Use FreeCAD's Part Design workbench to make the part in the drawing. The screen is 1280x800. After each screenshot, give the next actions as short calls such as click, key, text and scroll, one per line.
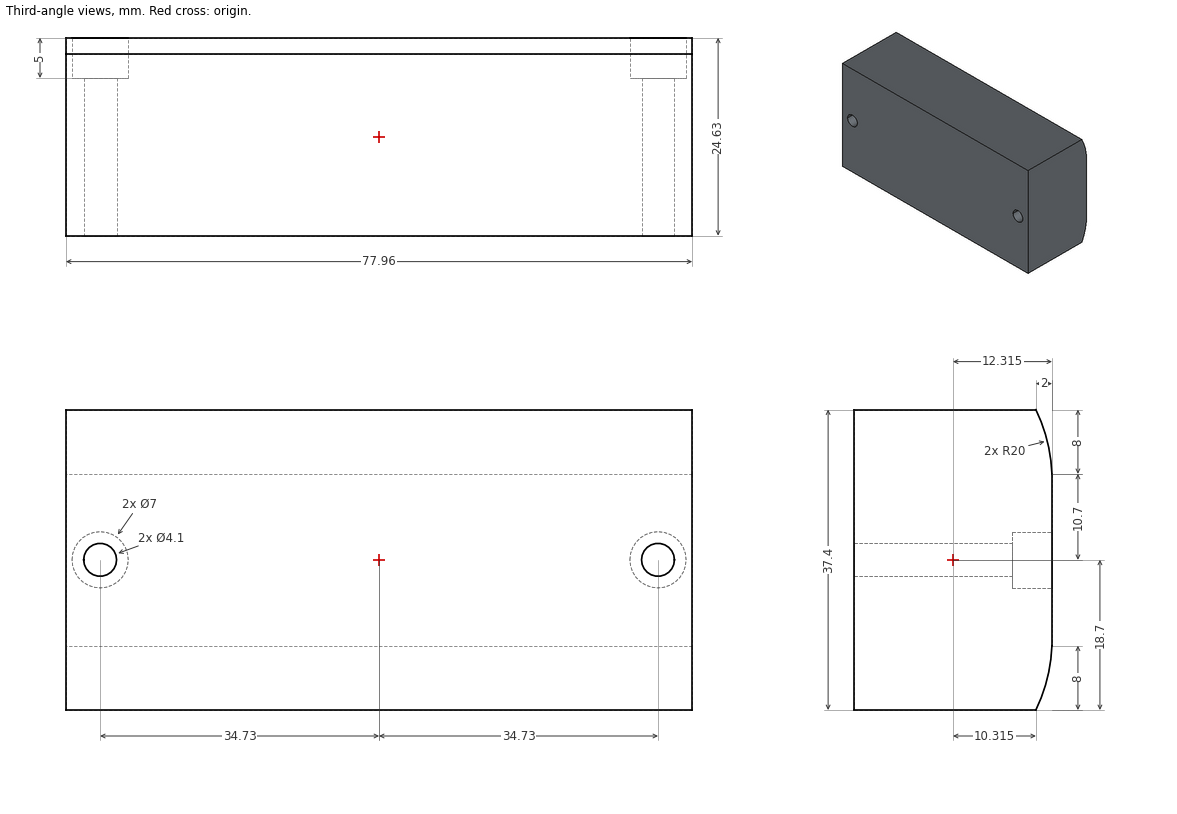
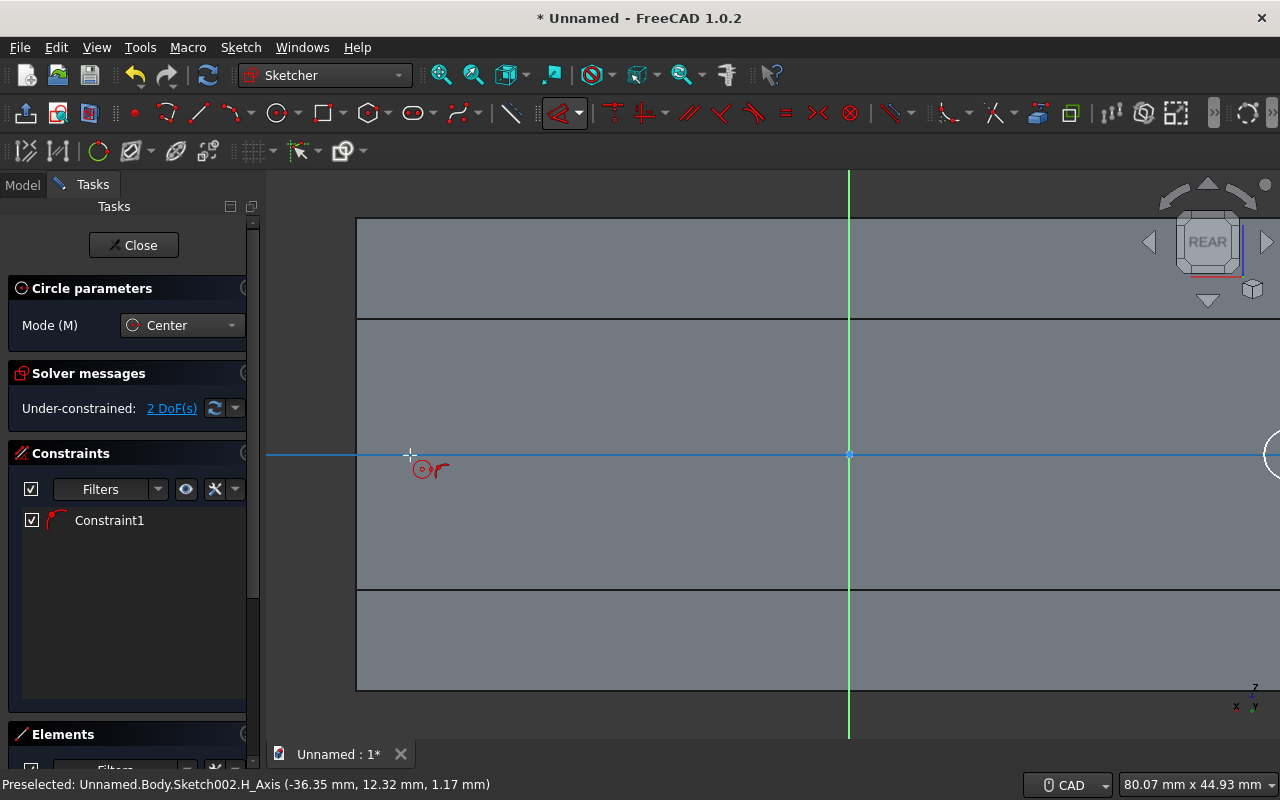
click(410, 454)
click(428, 436)
key(Escape)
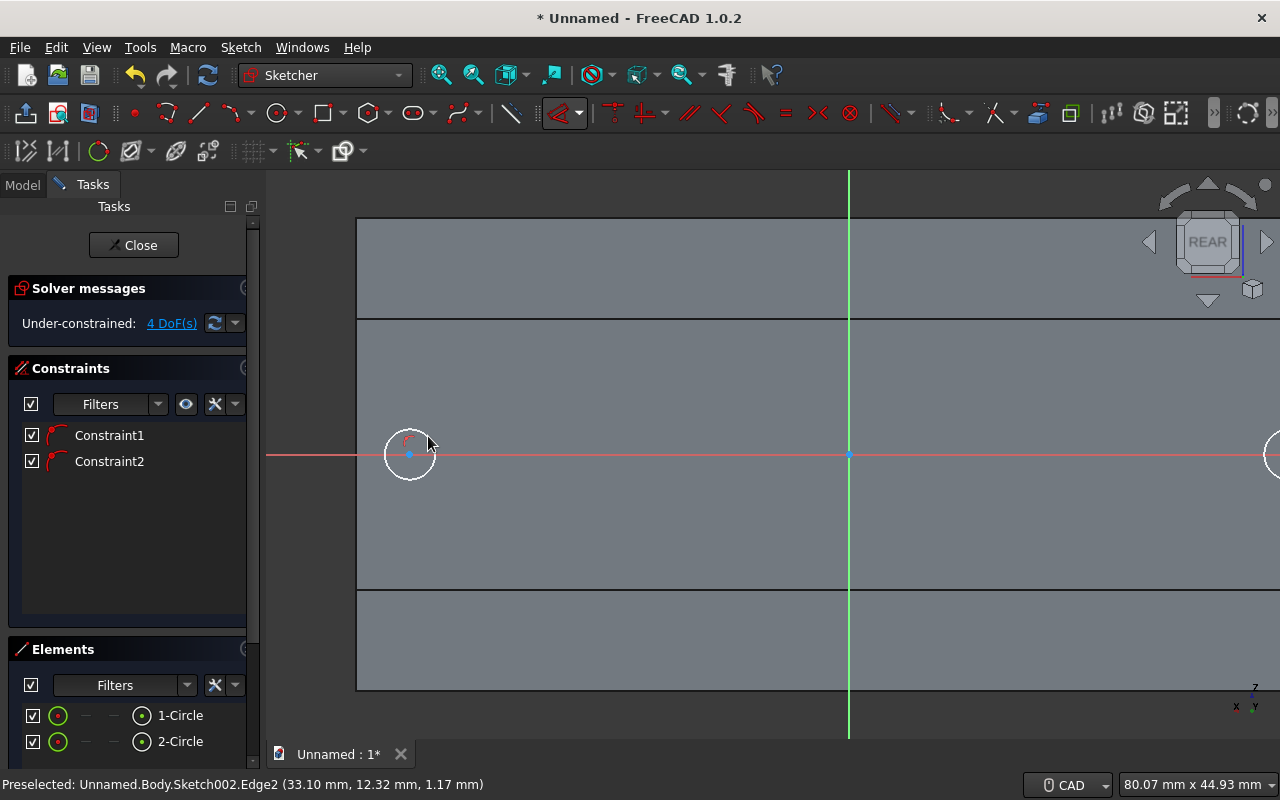
scroll(410, 455, down, 2)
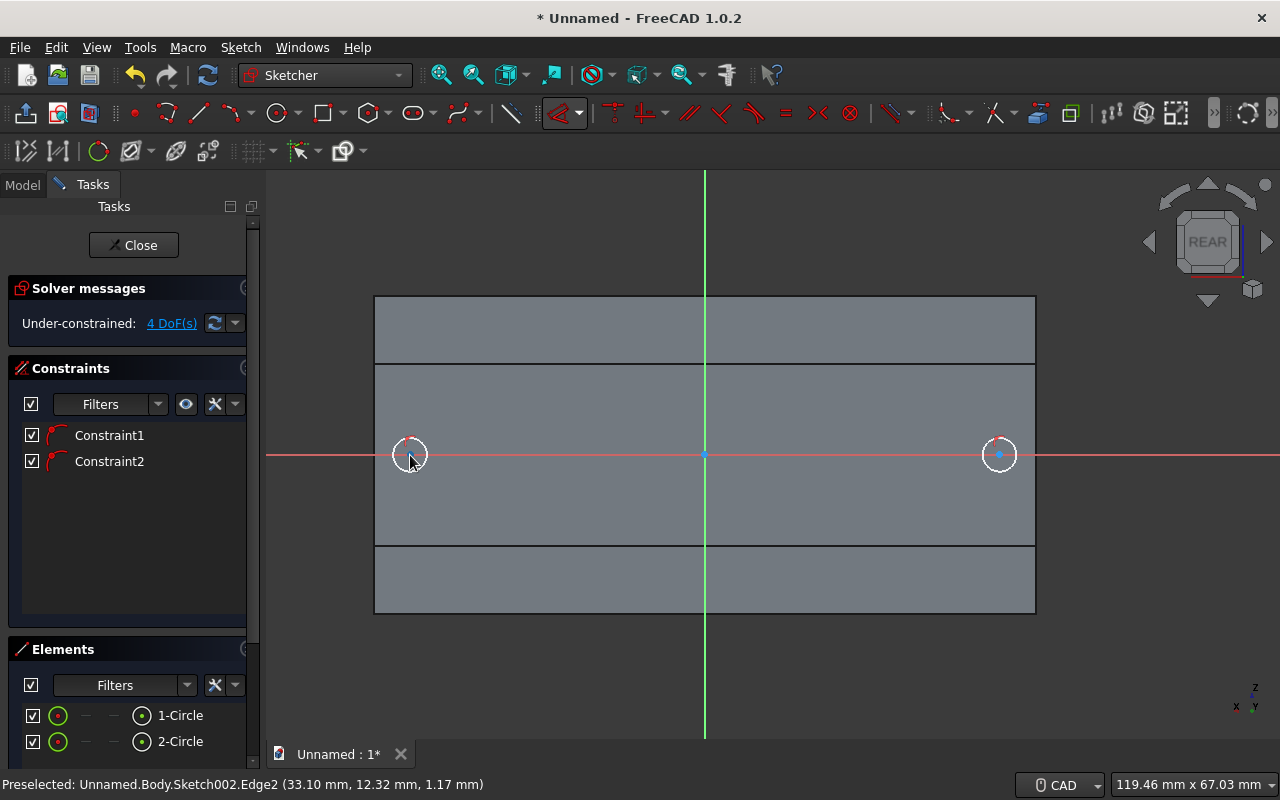
click(1011, 443)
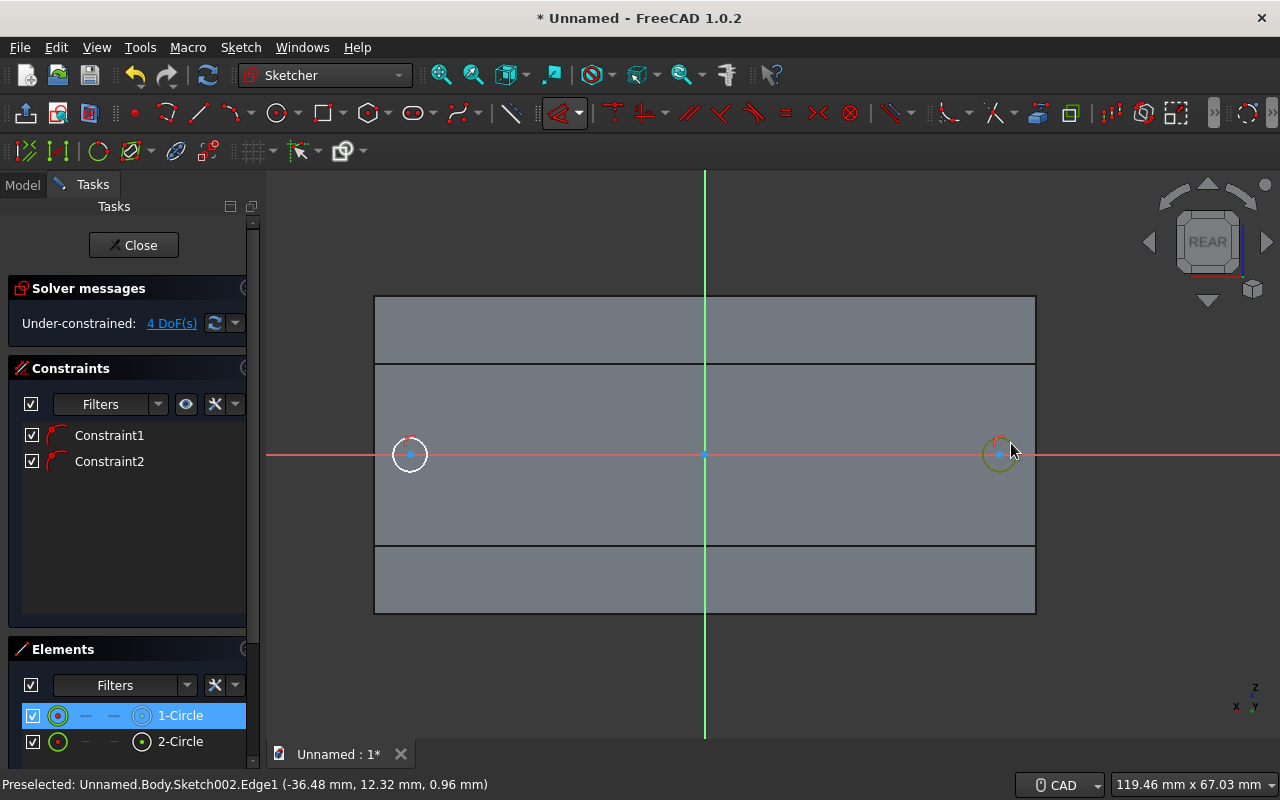
click(422, 443)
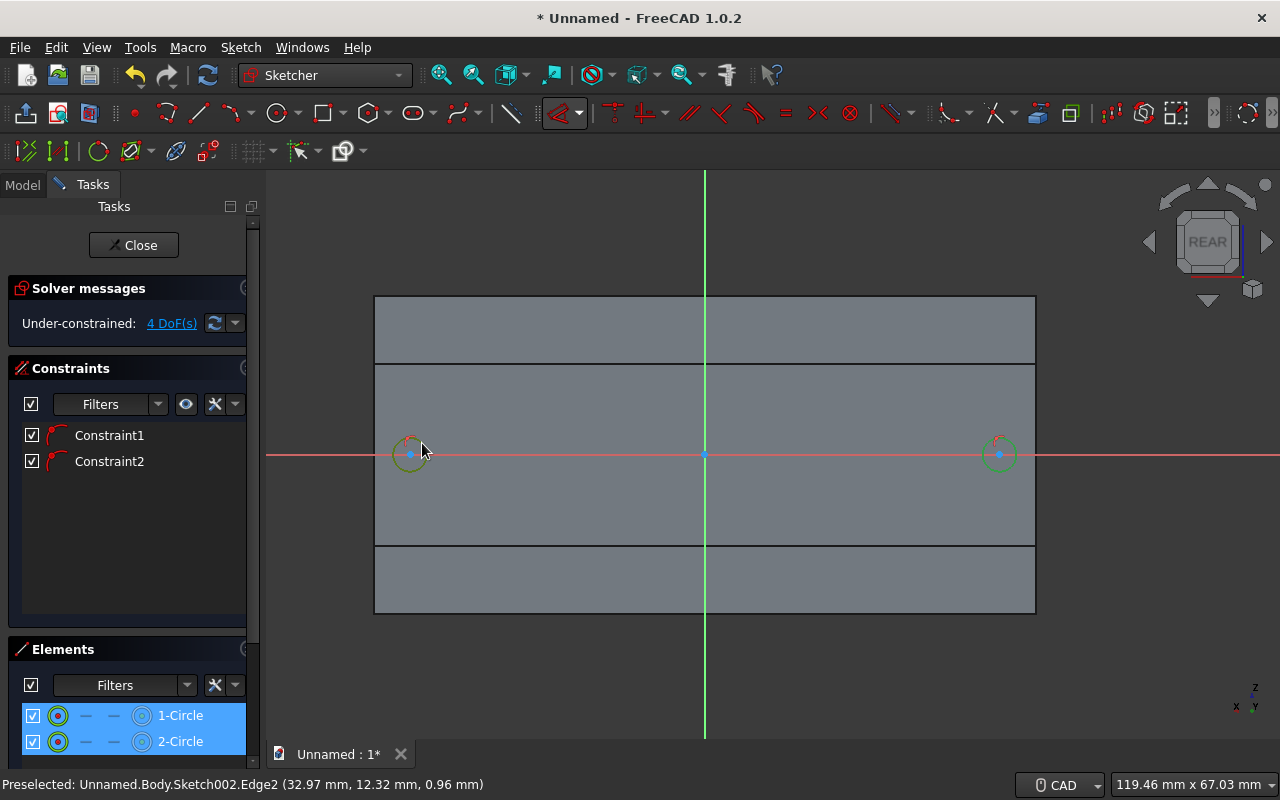
click(786, 114)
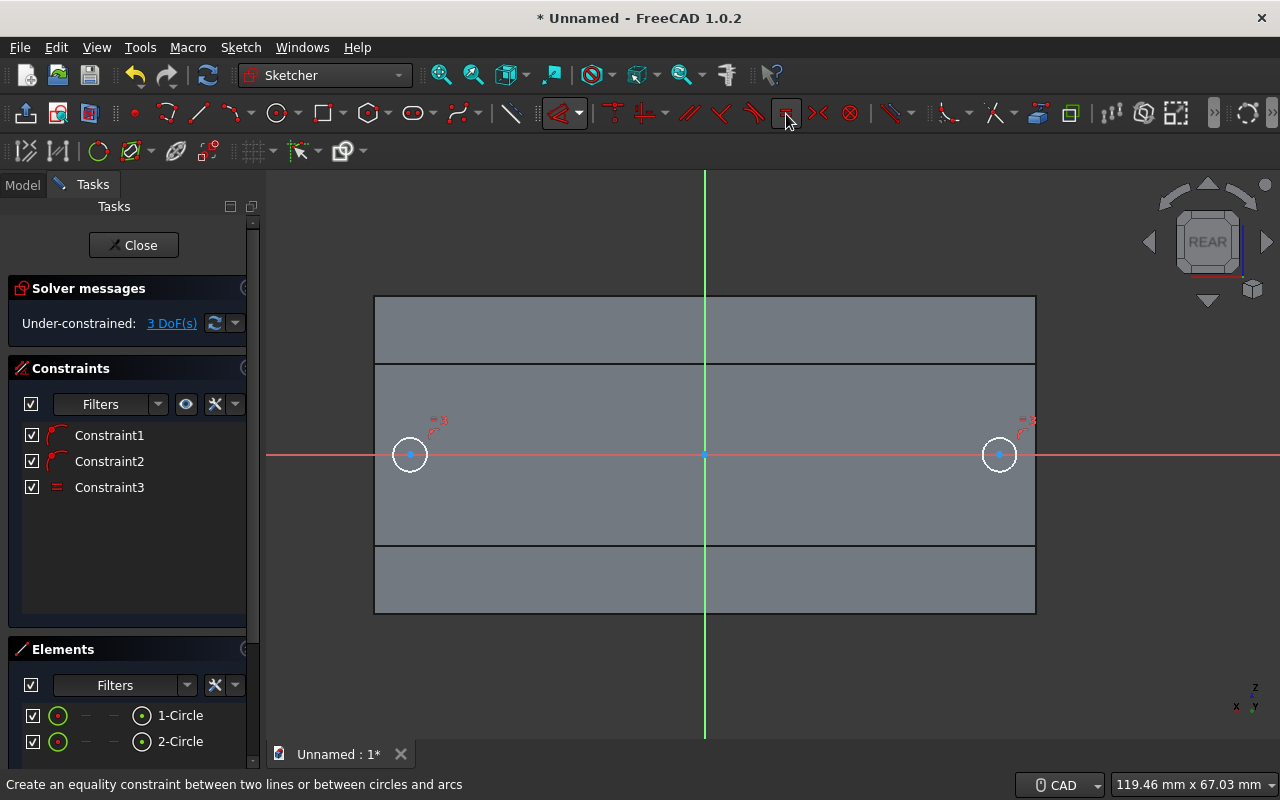
click(1011, 443)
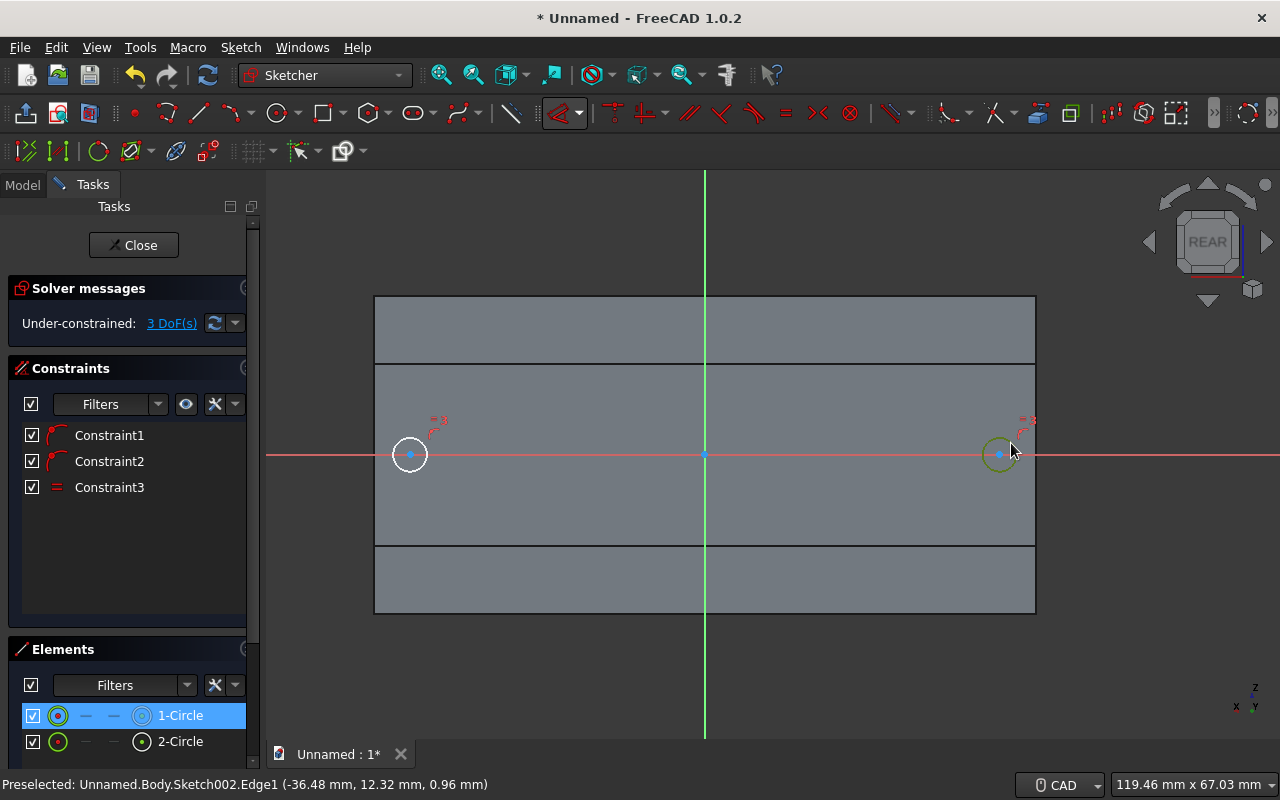
click(582, 114)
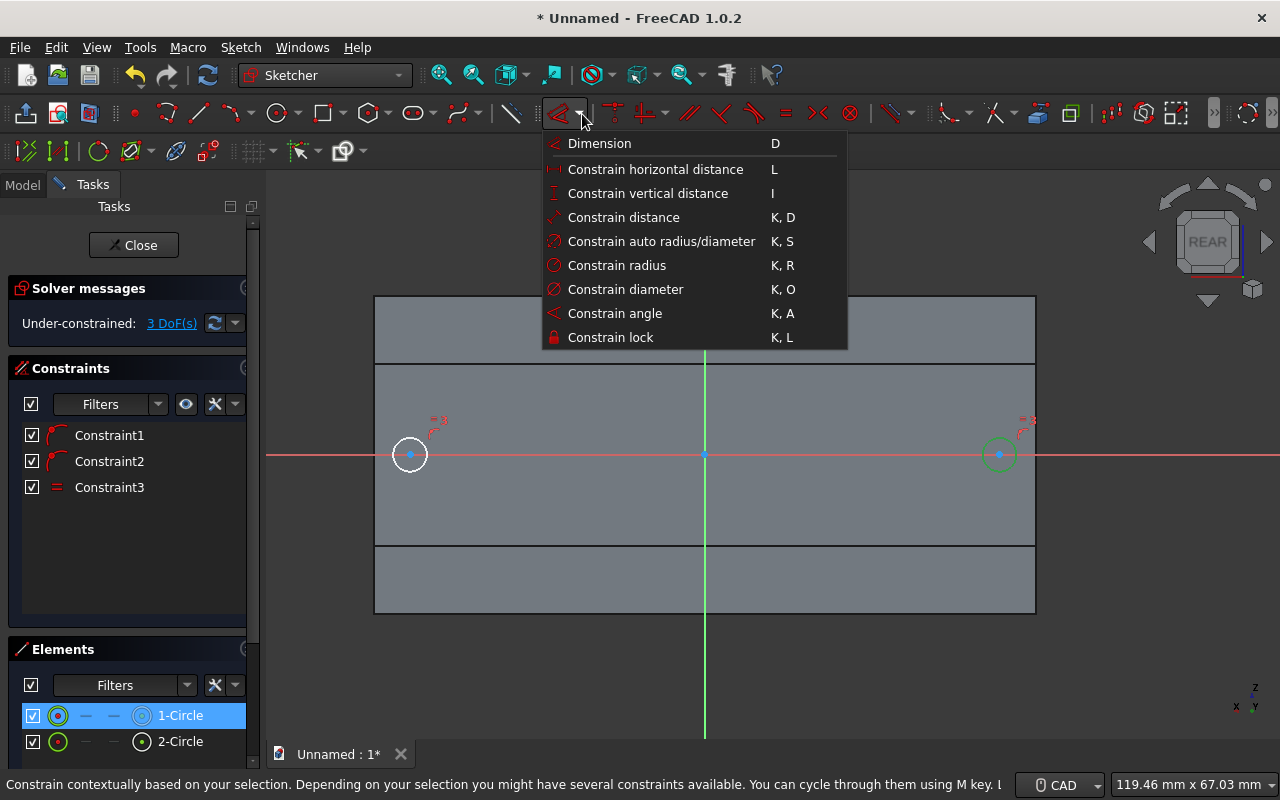
click(695, 289)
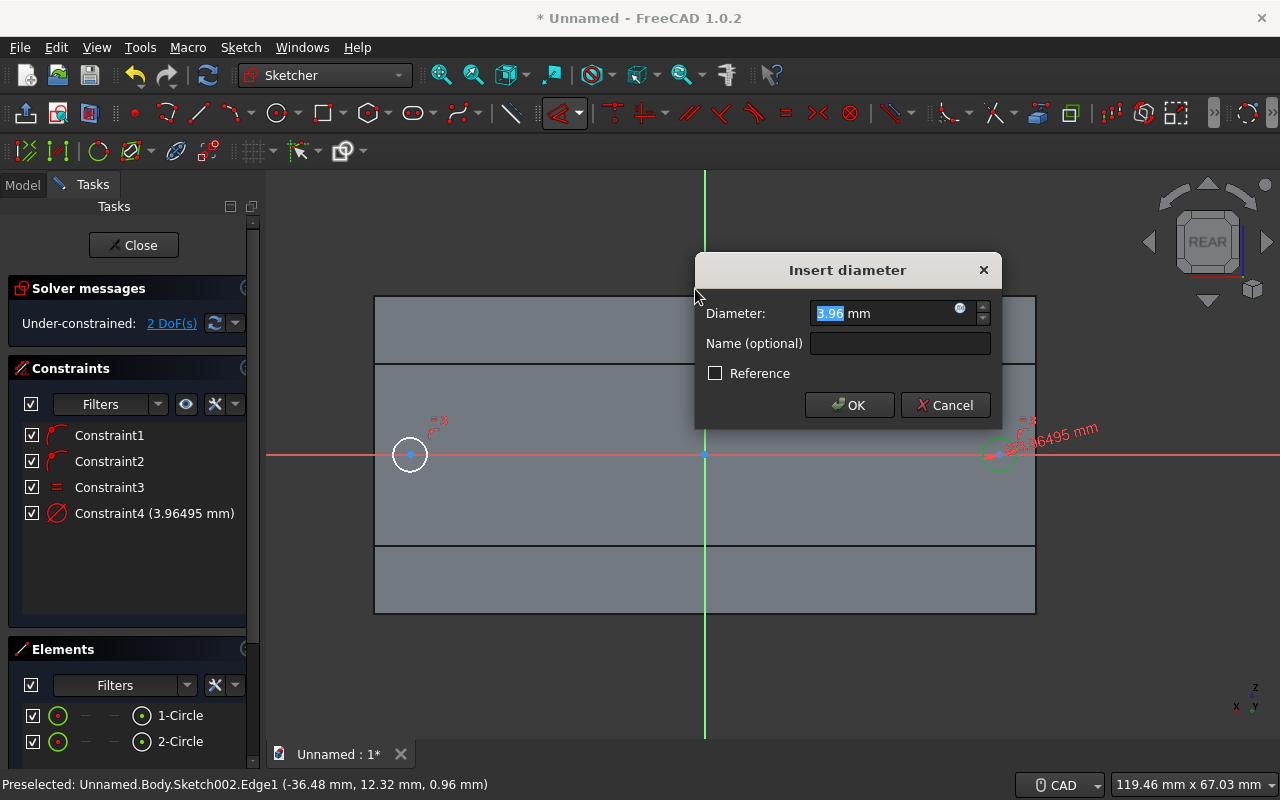
text(4.1)
key(Return)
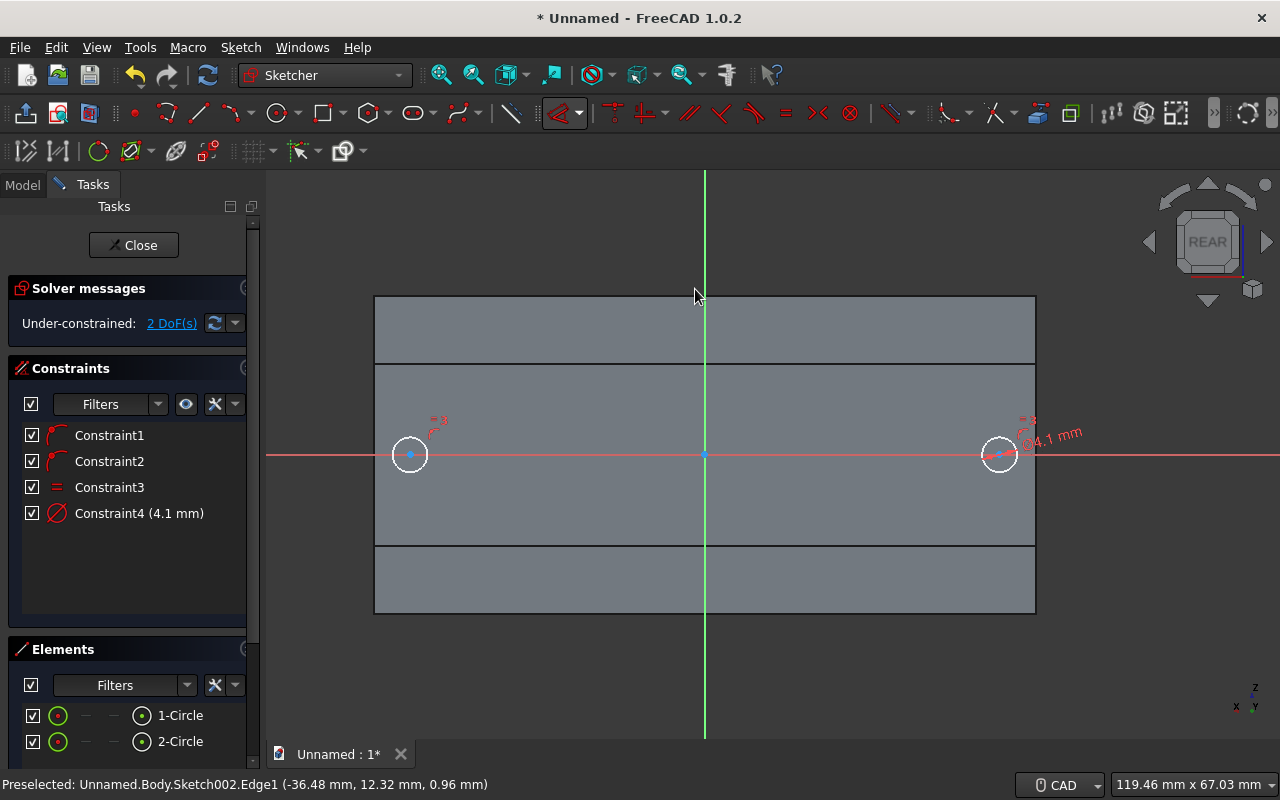
click(1000, 455)